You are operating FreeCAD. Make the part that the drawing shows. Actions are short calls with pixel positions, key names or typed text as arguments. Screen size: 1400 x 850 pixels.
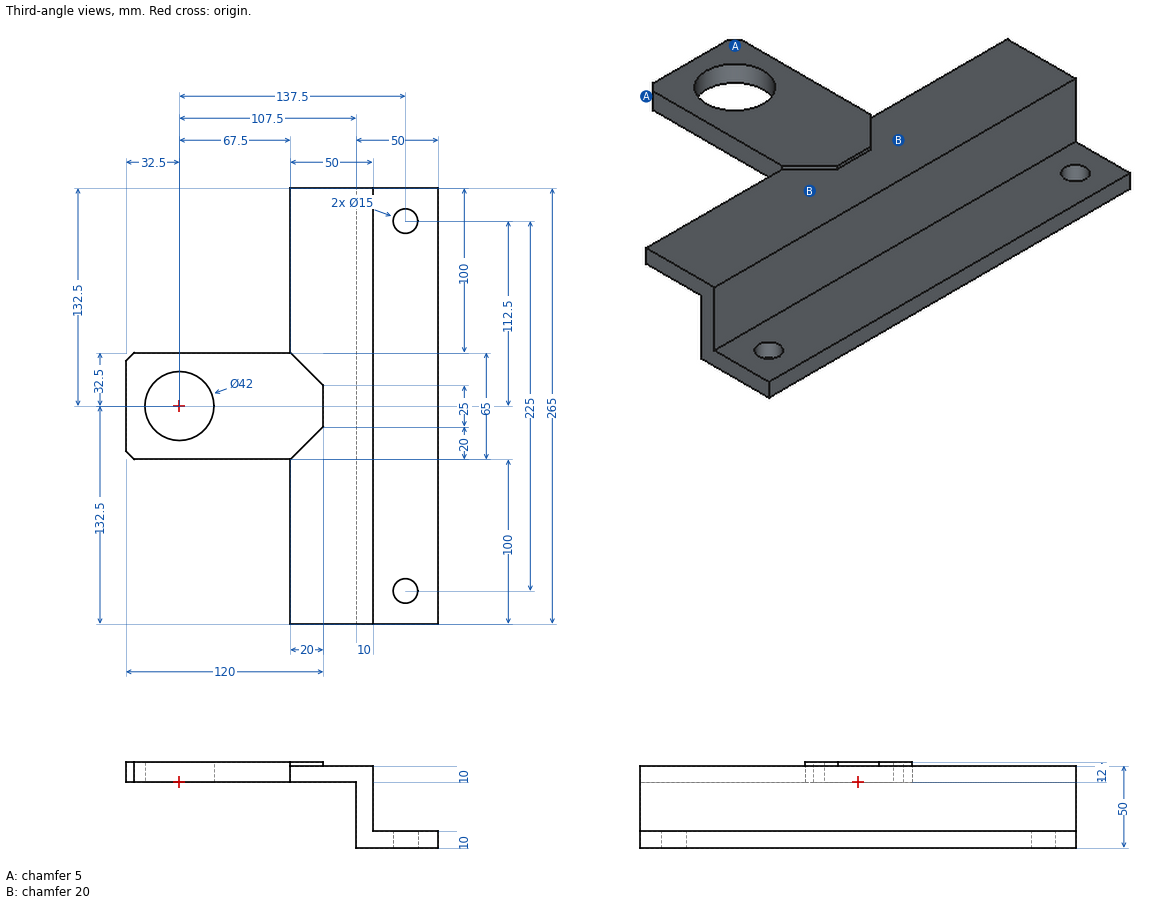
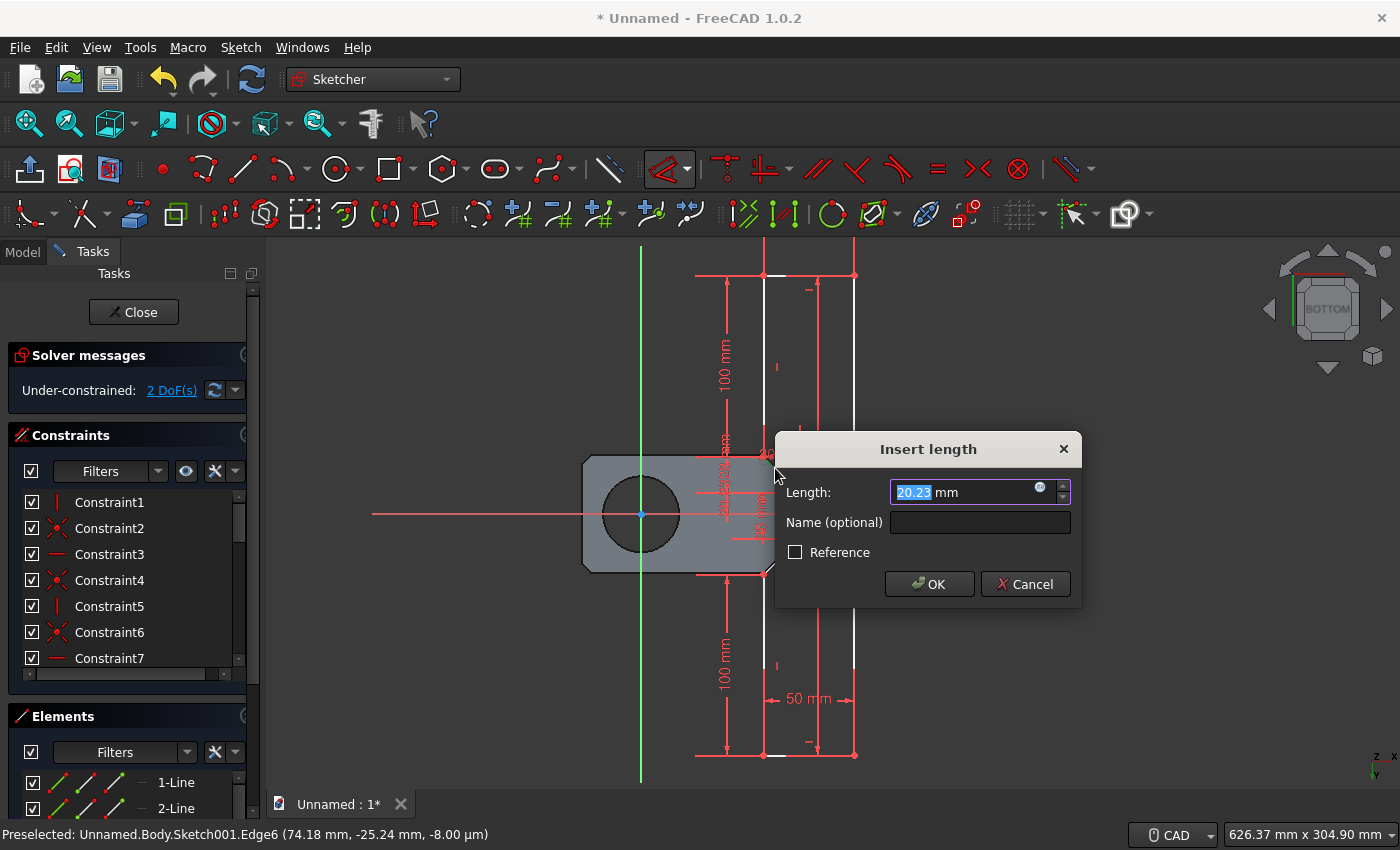
text(20)
key(Return)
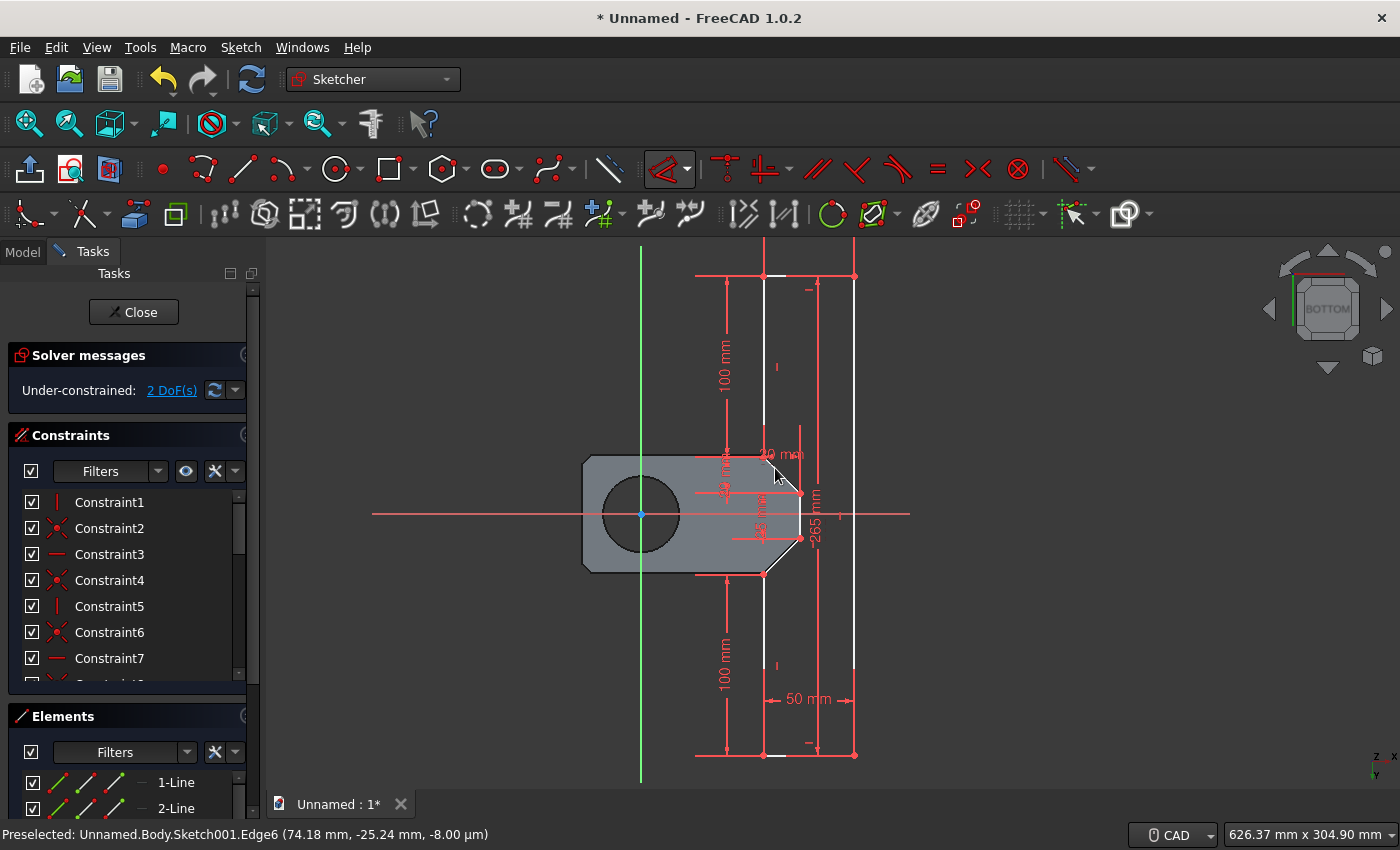
click(764, 575)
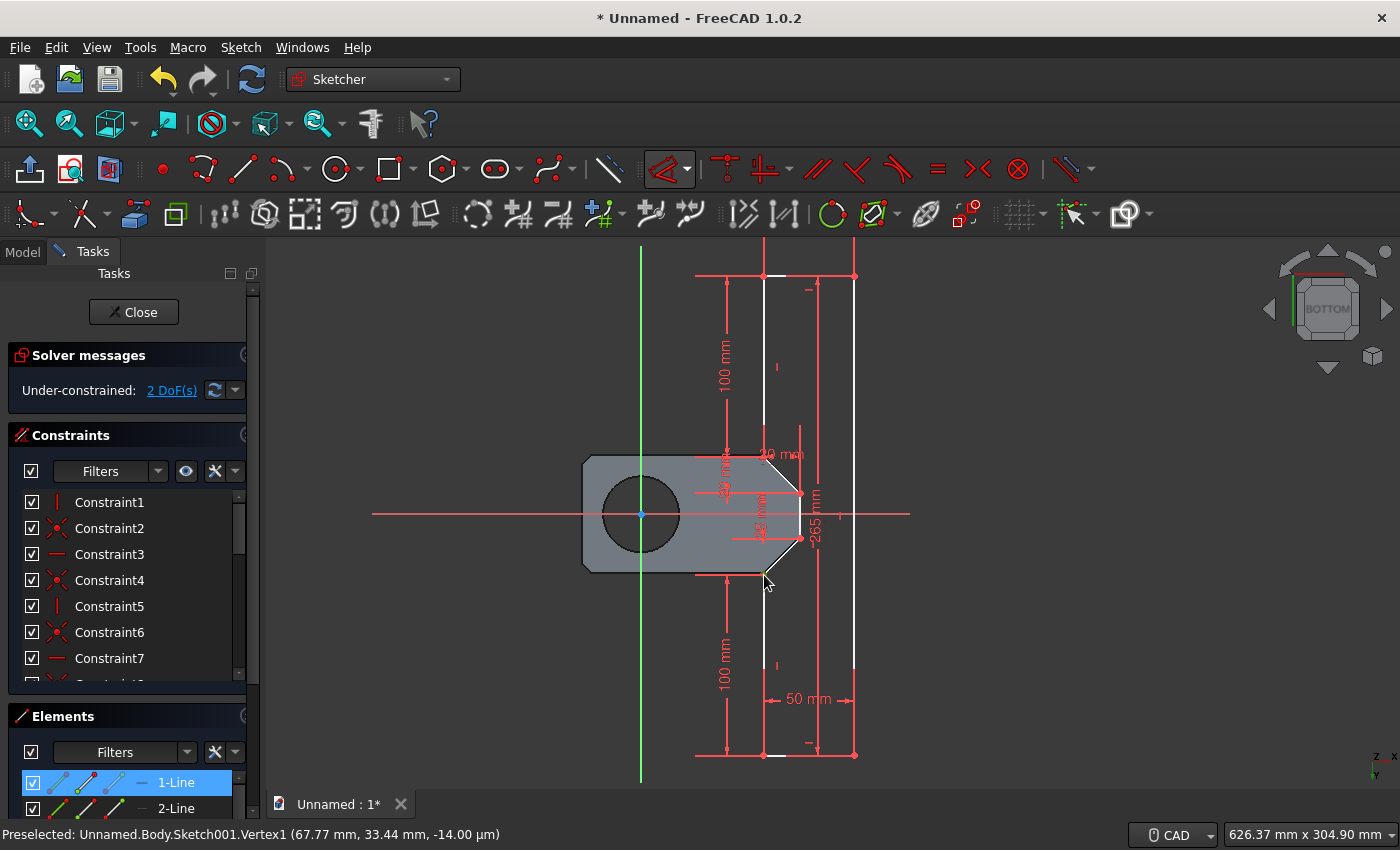
key(l)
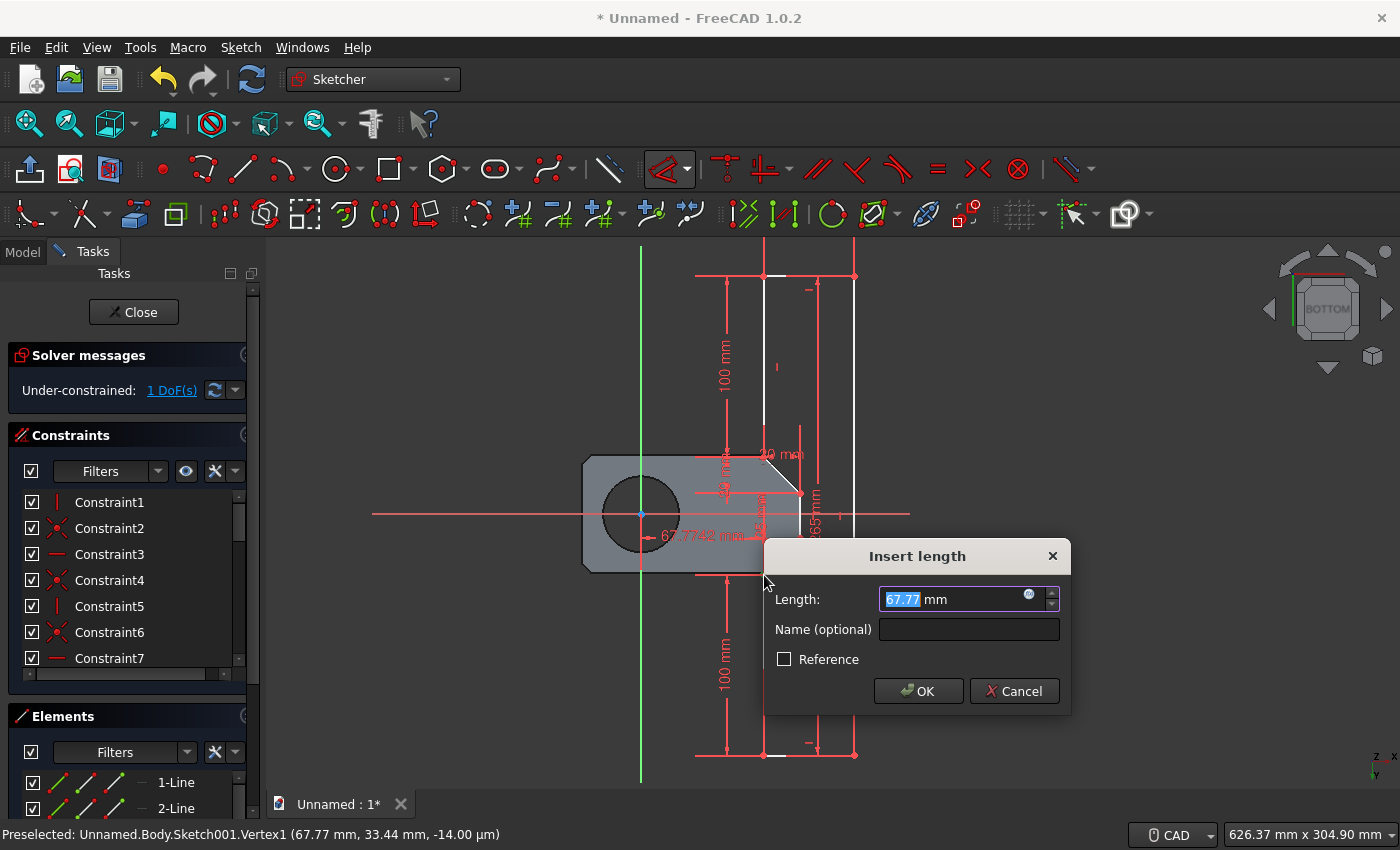
text(67.5)
key(Return)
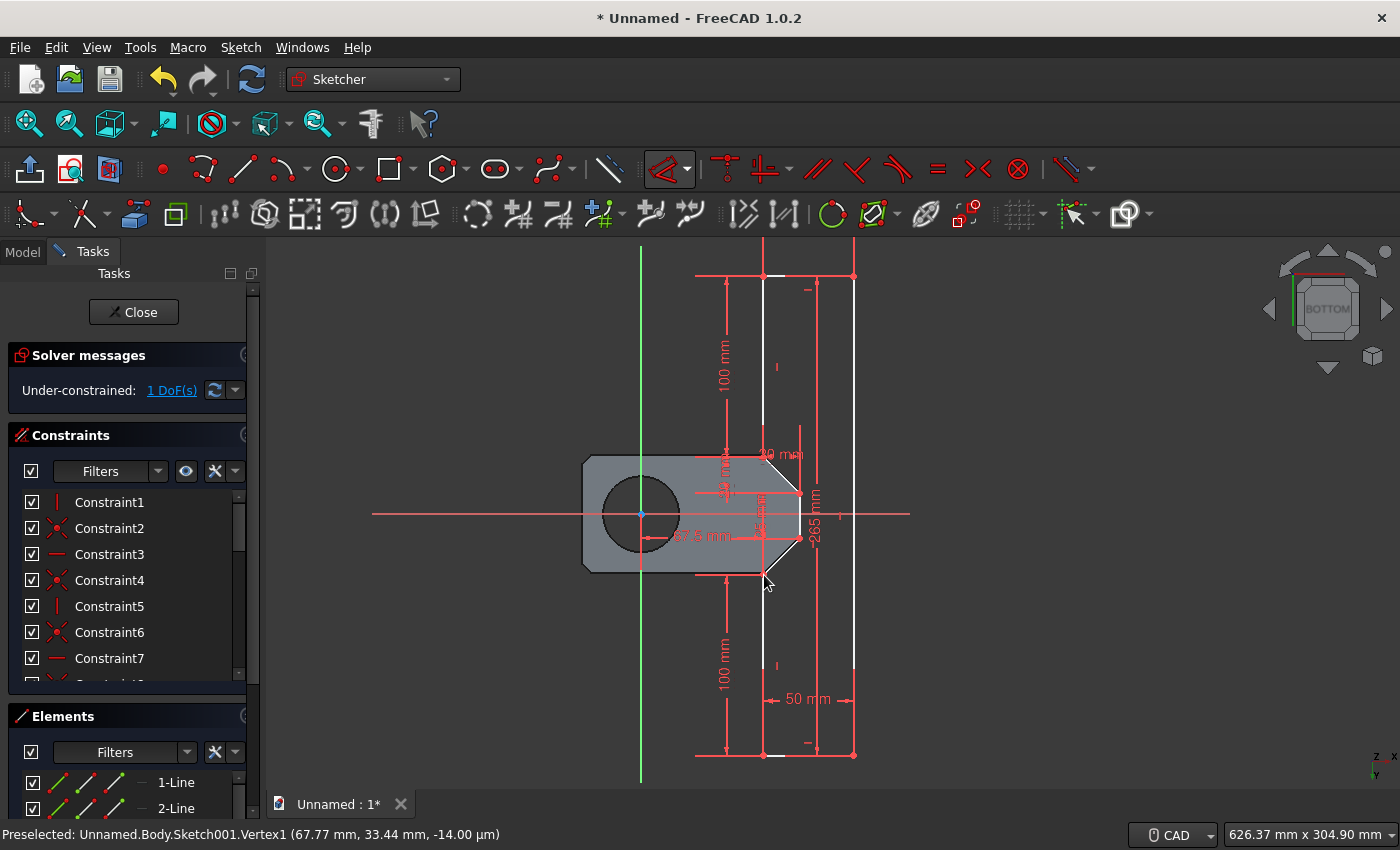
click(763, 575)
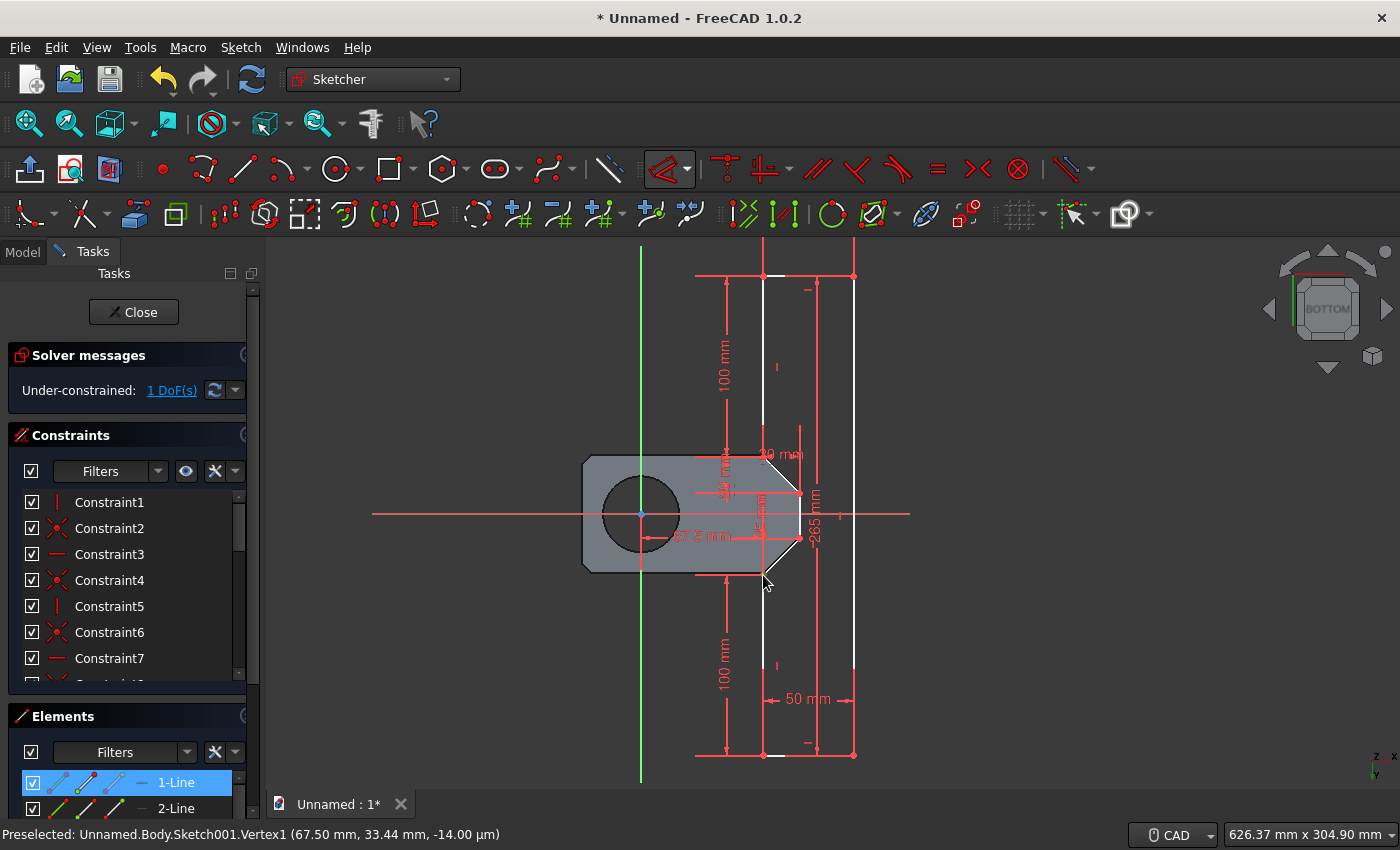
key(i)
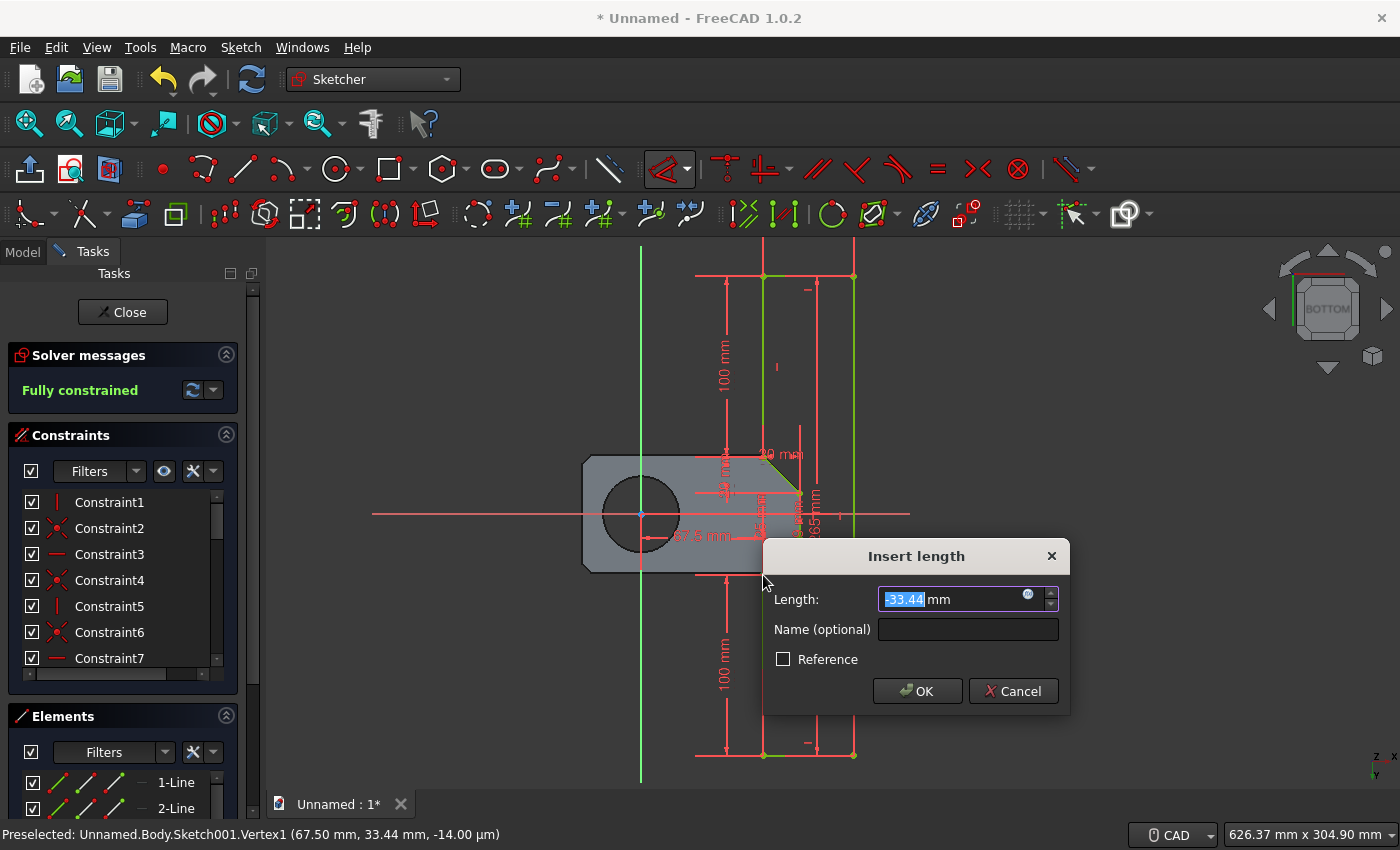
text(-32.5)
key(Return)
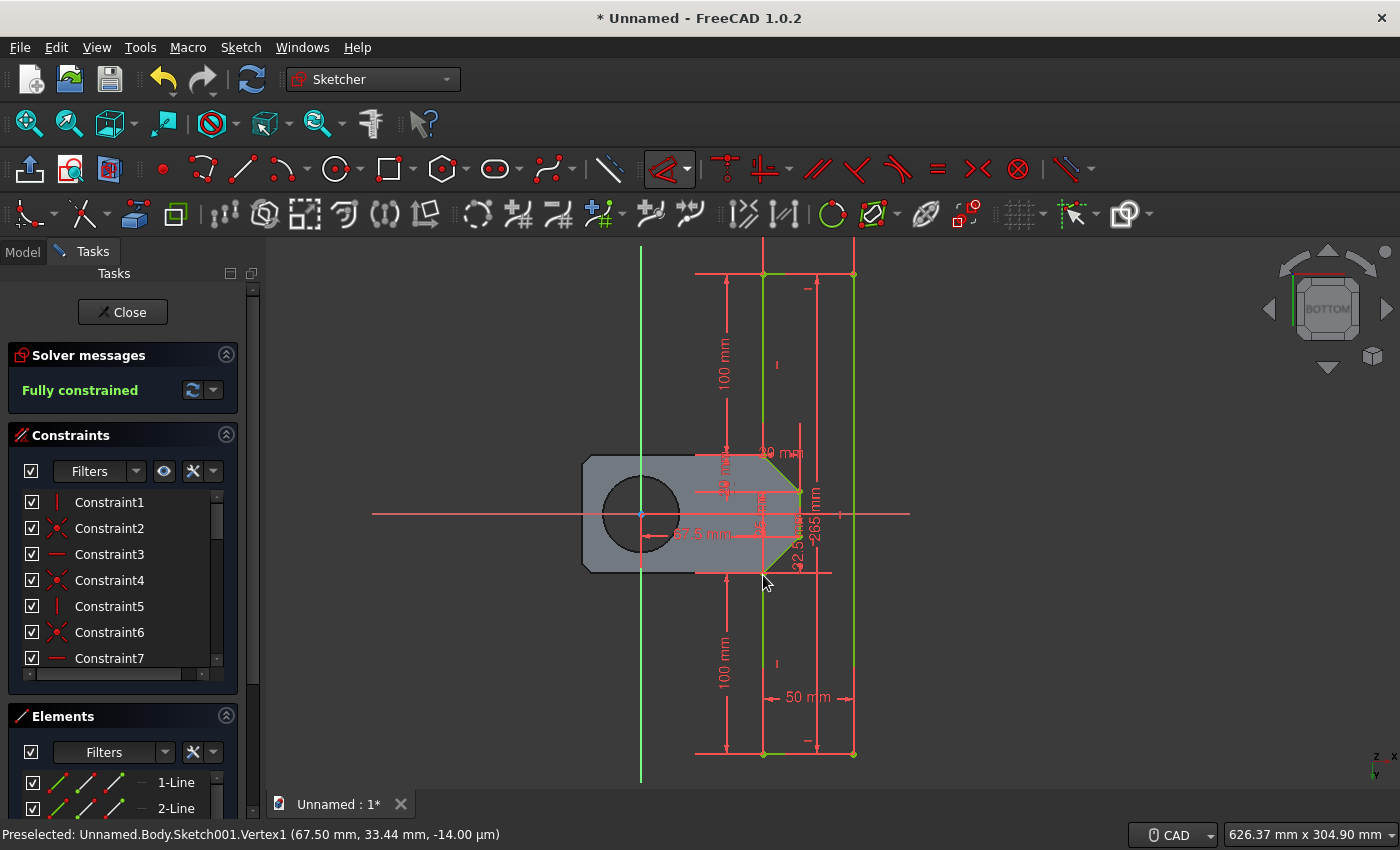
click(123, 312)